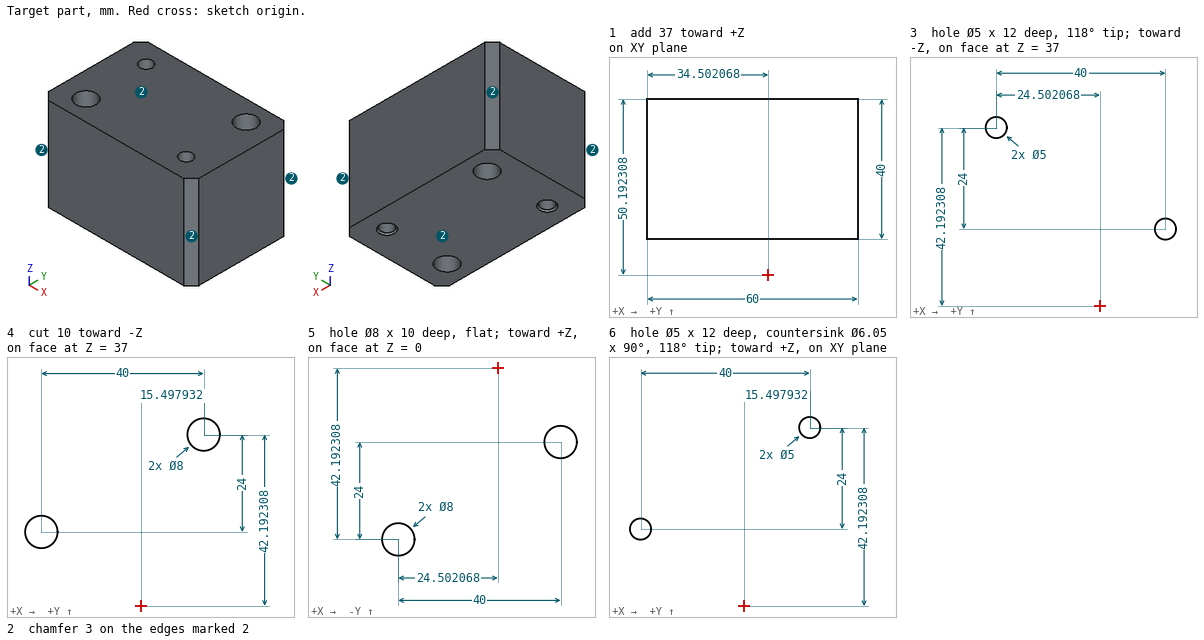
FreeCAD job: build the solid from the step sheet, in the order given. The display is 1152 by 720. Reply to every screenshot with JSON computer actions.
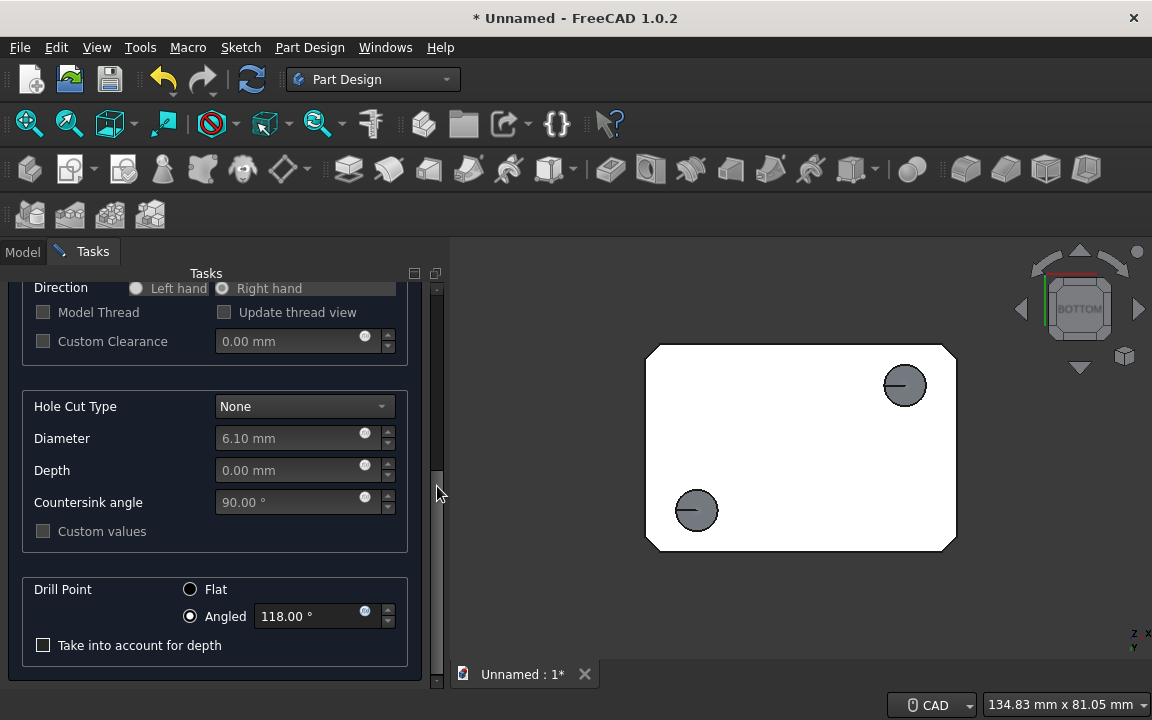
{"action": "left_click", "coordinate": [191, 589]}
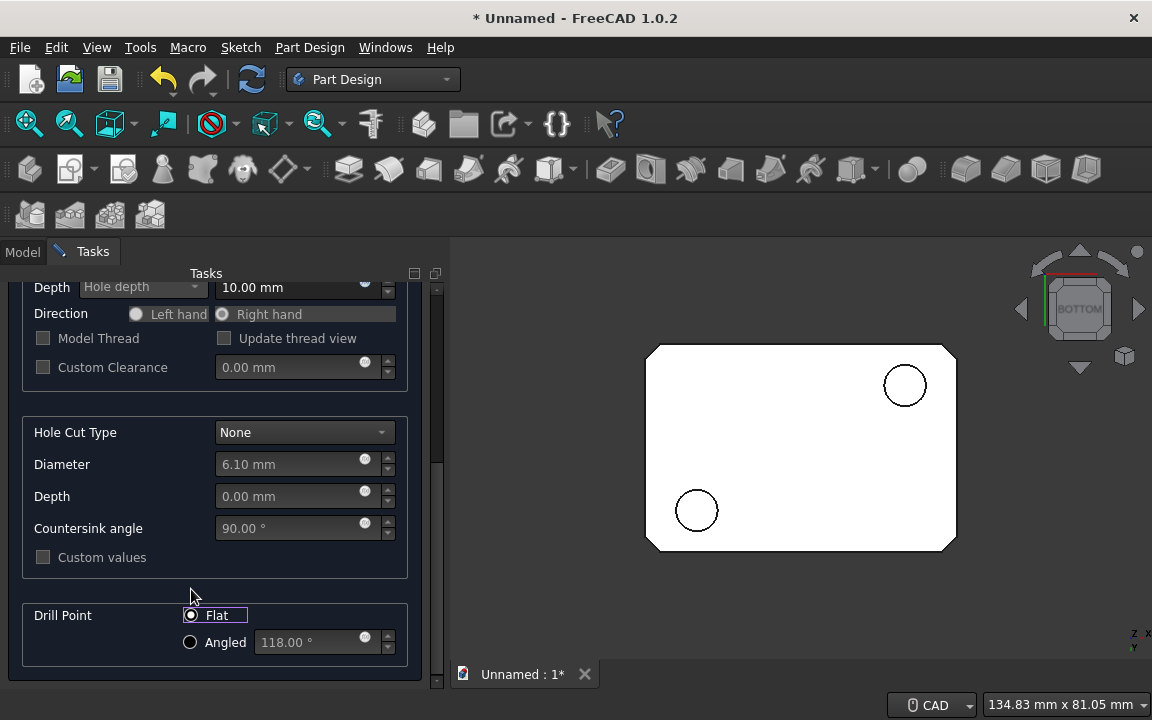
{"action": "scroll", "coordinate": [437, 486], "scroll_direction": "up", "scroll_amount": 7}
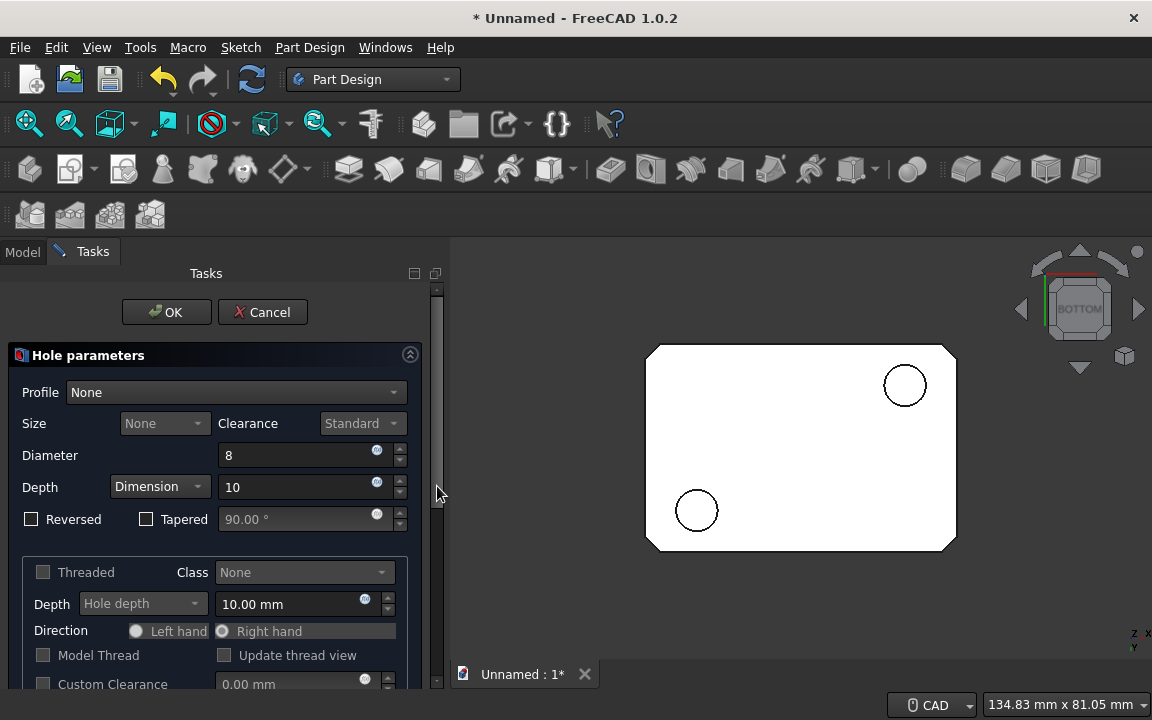
{"action": "left_click", "coordinate": [167, 312]}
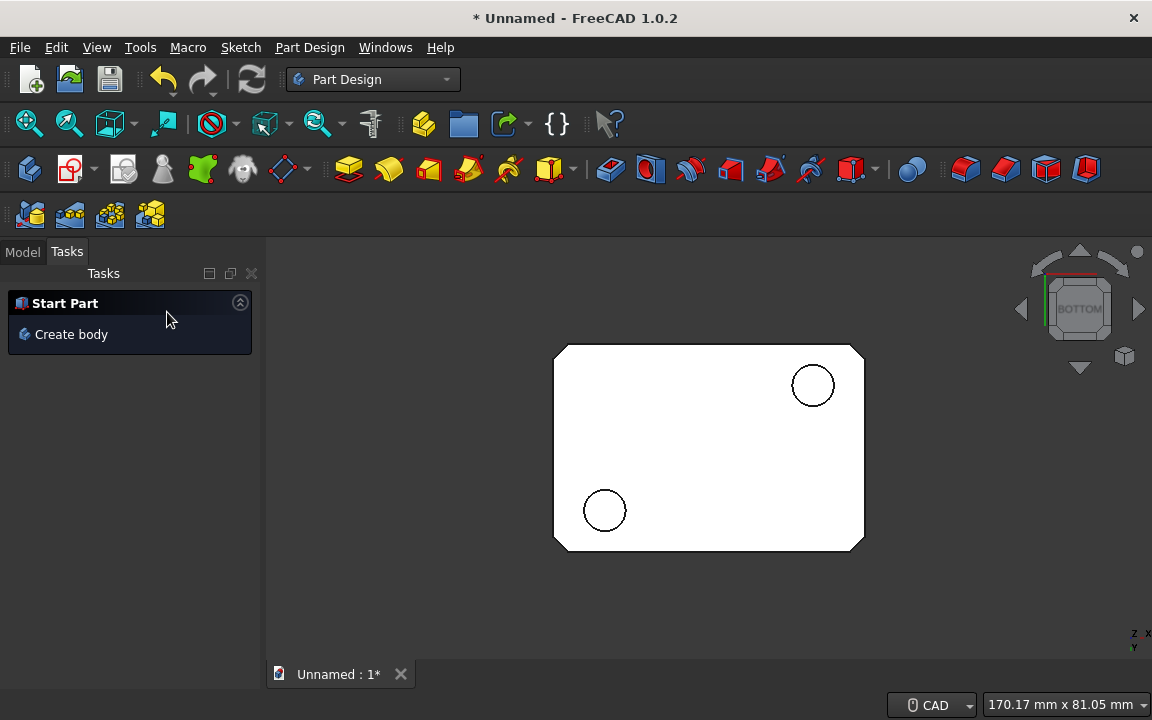
{"action": "left_click", "coordinate": [70, 170]}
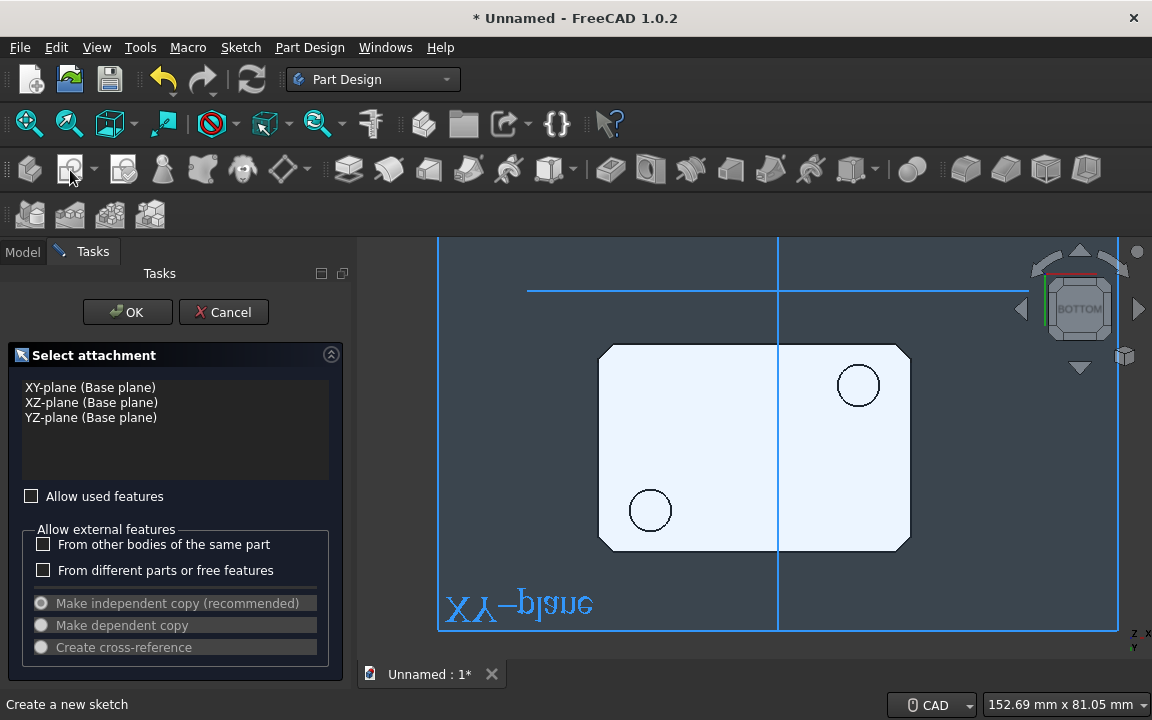
{"action": "left_click", "coordinate": [82, 388]}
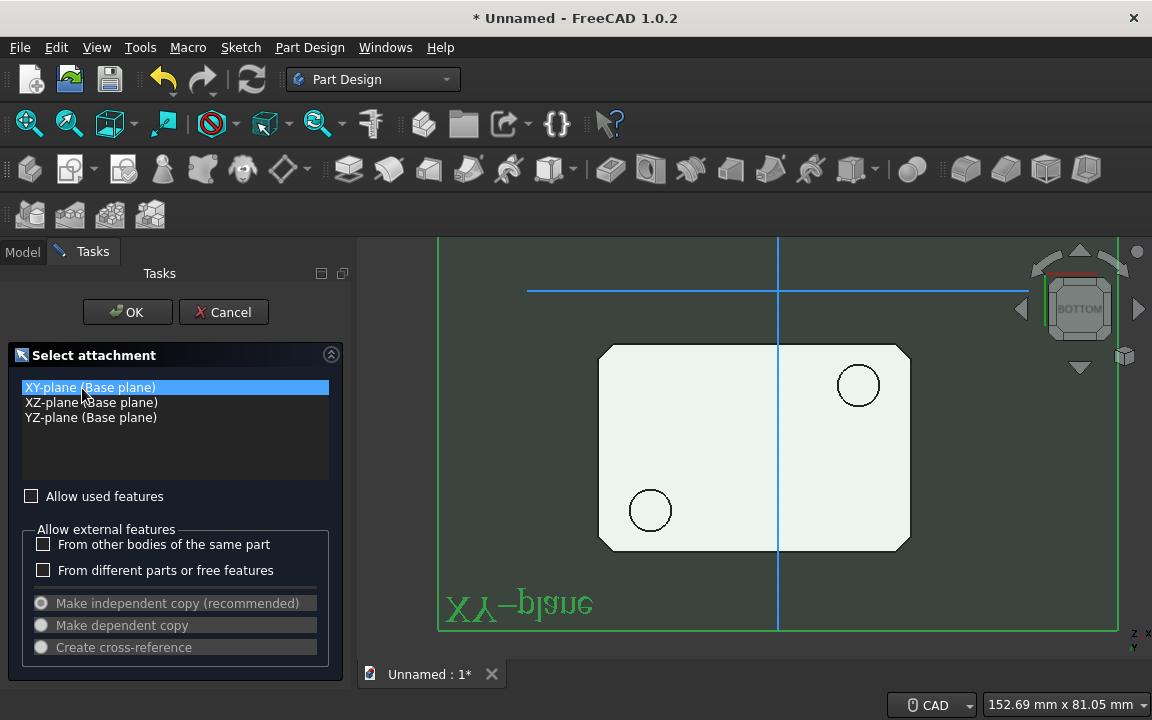
{"action": "left_click", "coordinate": [128, 312]}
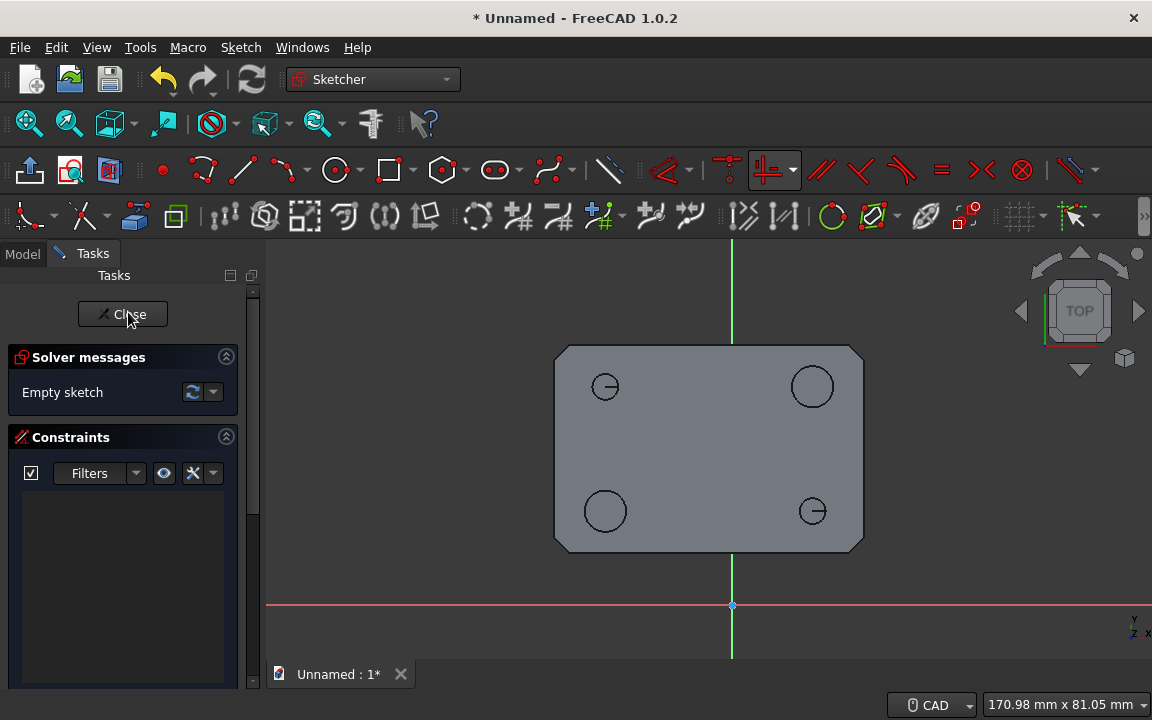
{"action": "left_click", "coordinate": [110, 170]}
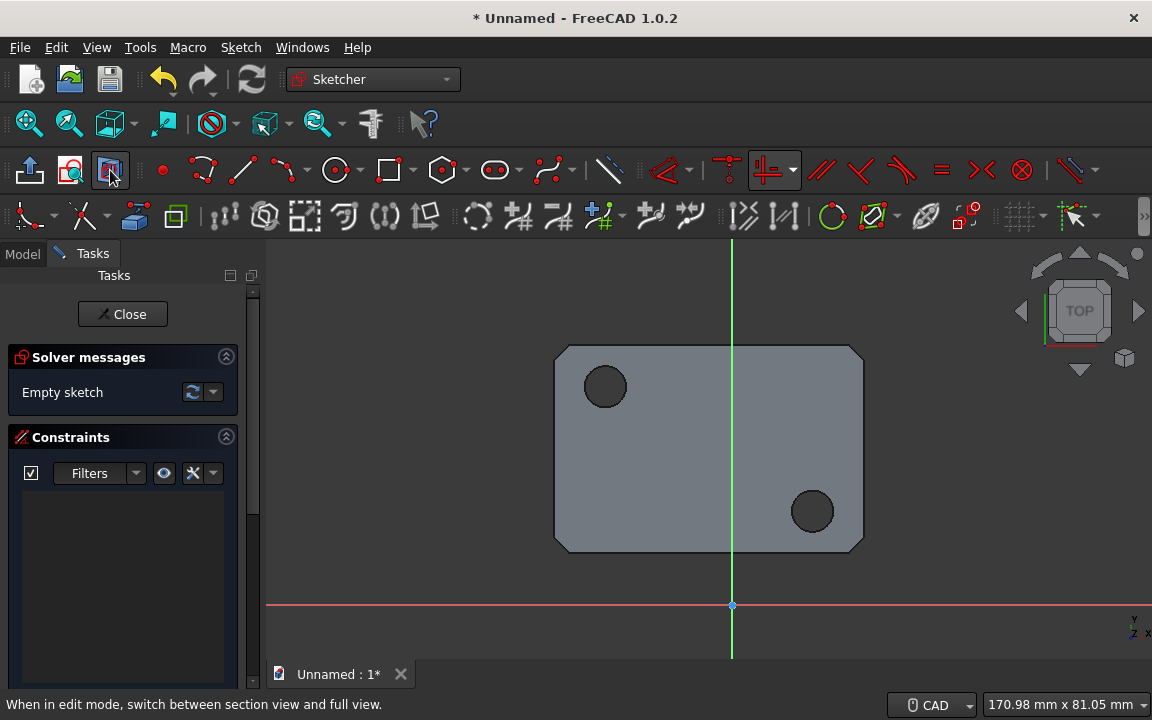
{"action": "left_click", "coordinate": [336, 170]}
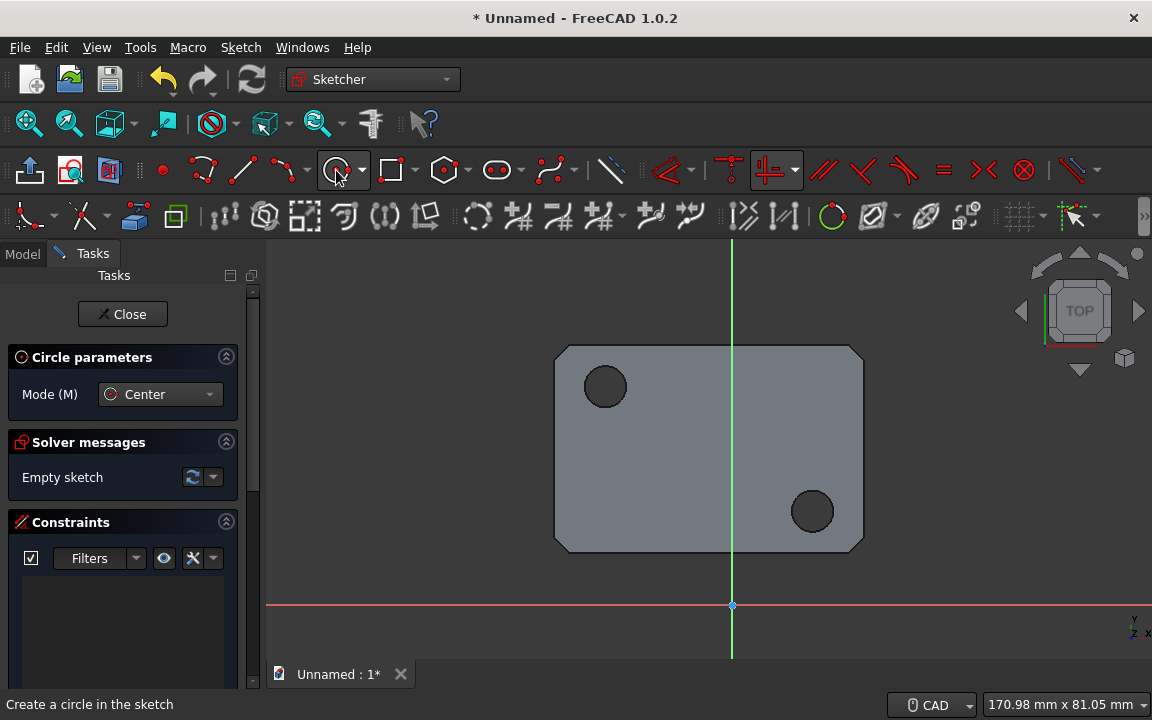
{"action": "scroll", "coordinate": [813, 387], "scroll_direction": "up", "scroll_amount": 3}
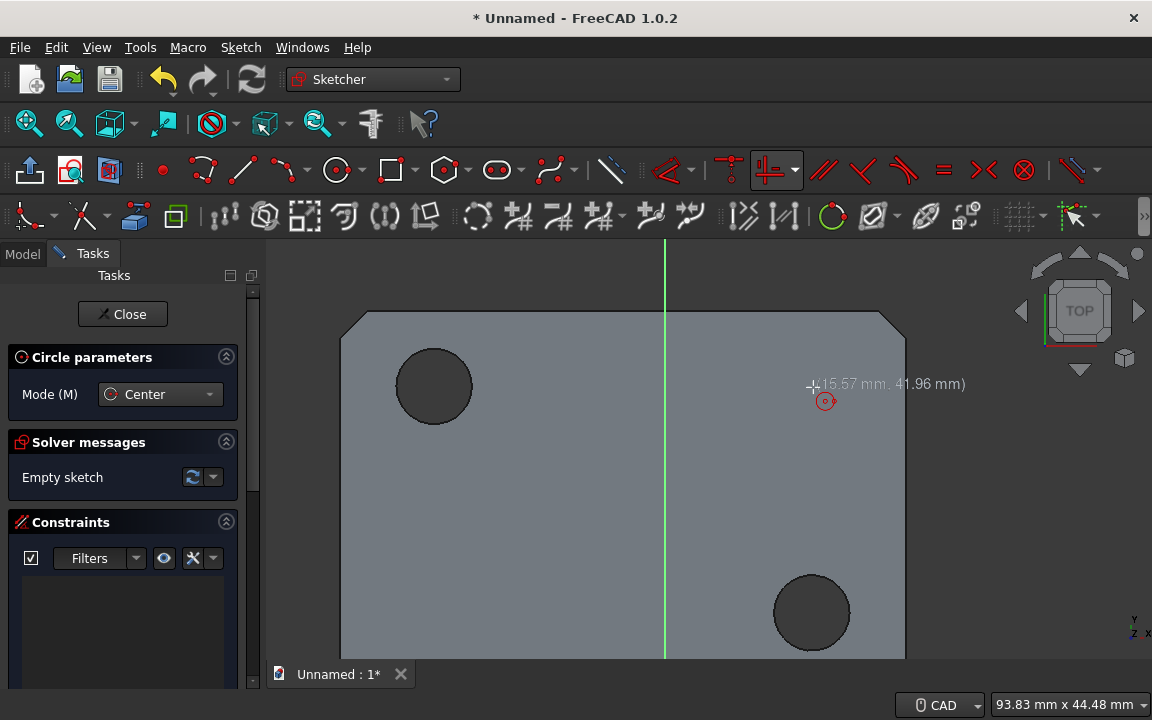
{"action": "left_click", "coordinate": [812, 386]}
{"action": "mouse_move", "coordinate": [829, 370]}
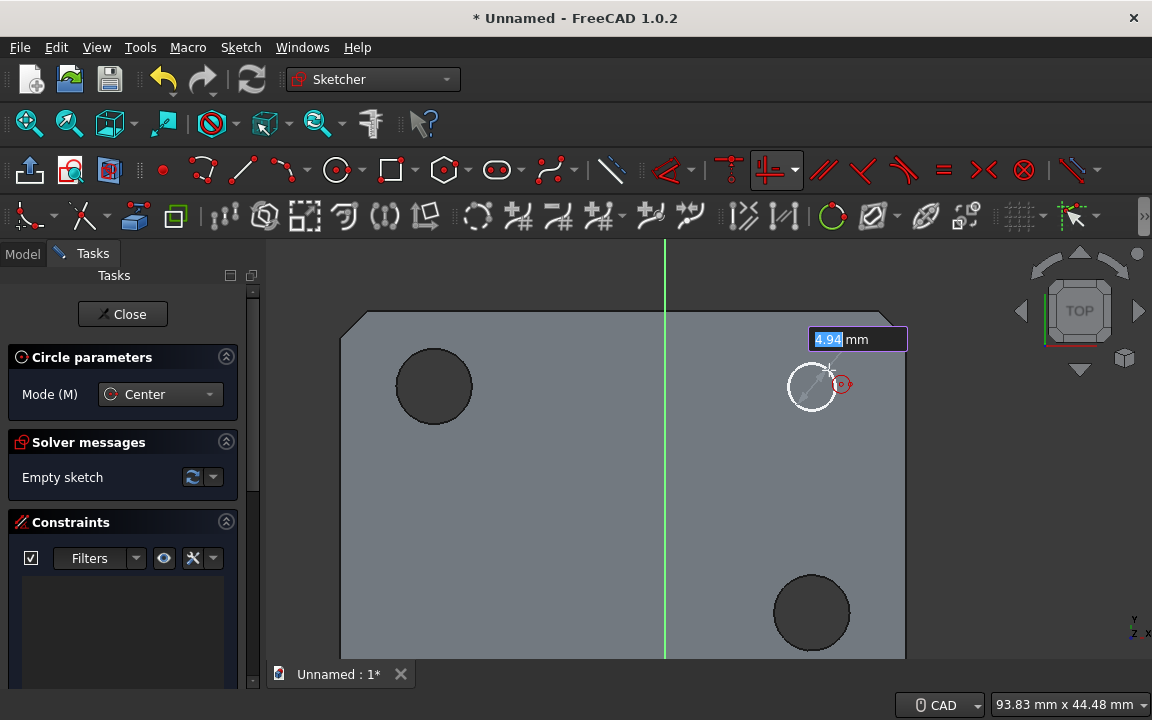
{"action": "type", "text": "5"}
{"action": "key", "text": "Return"}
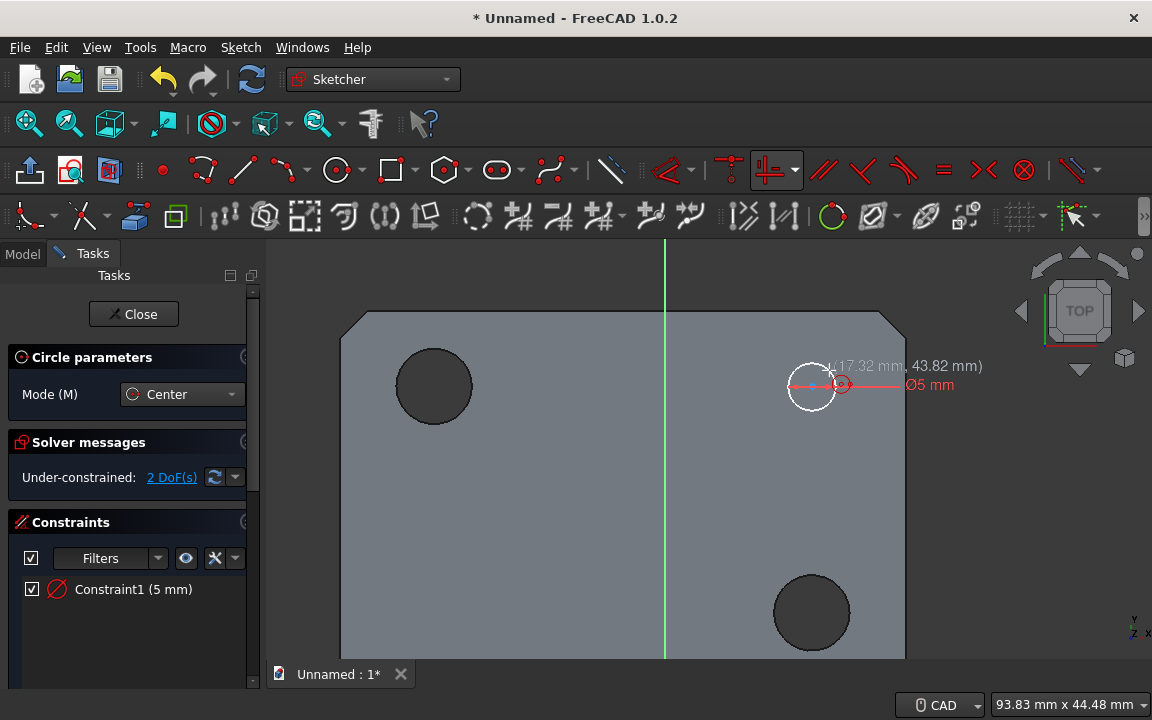
{"action": "left_click", "coordinate": [434, 613]}
{"action": "mouse_move", "coordinate": [451, 596]}